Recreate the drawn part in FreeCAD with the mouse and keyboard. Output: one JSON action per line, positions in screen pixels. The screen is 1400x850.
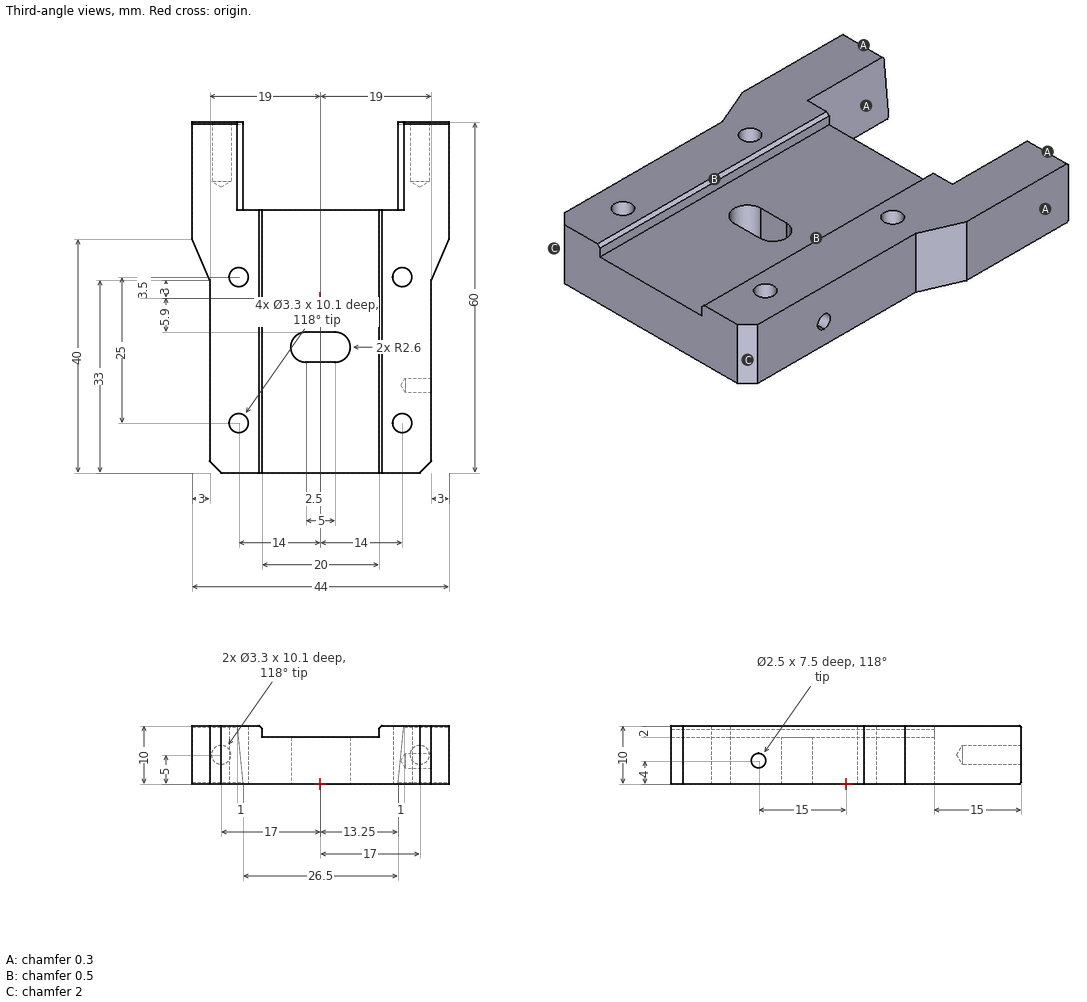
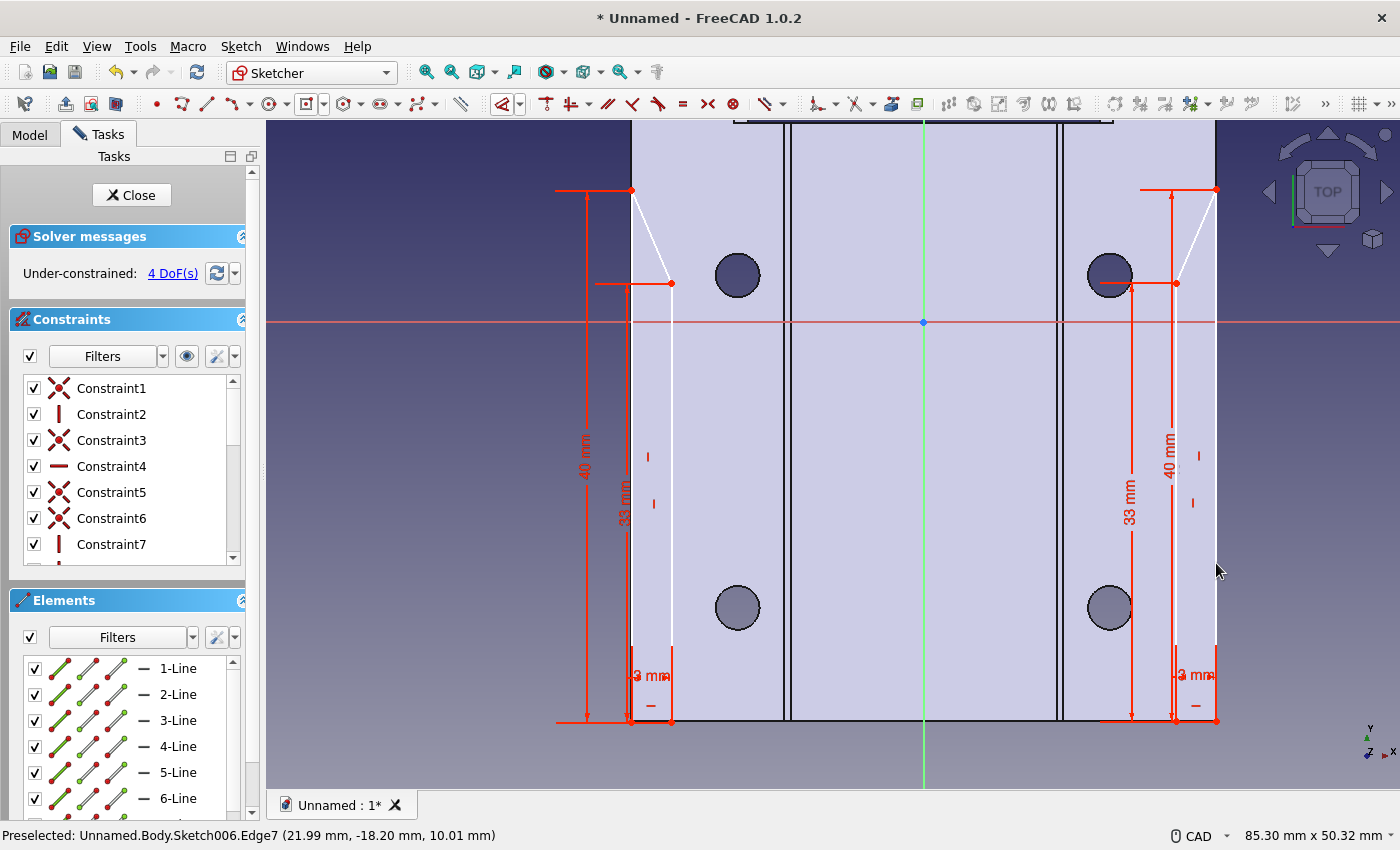
{"action": "left_click", "coordinate": [672, 284]}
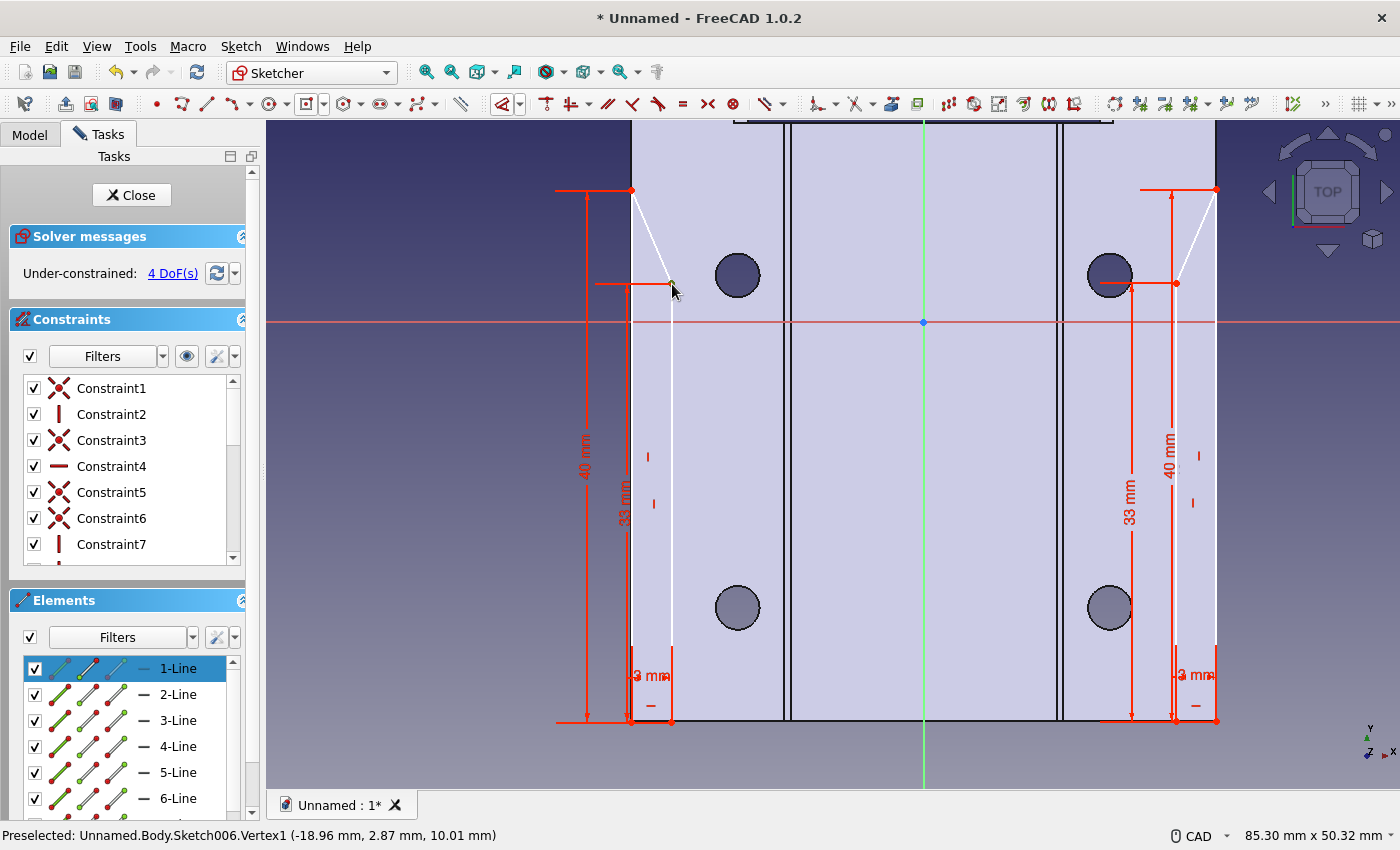
{"action": "key", "text": "i"}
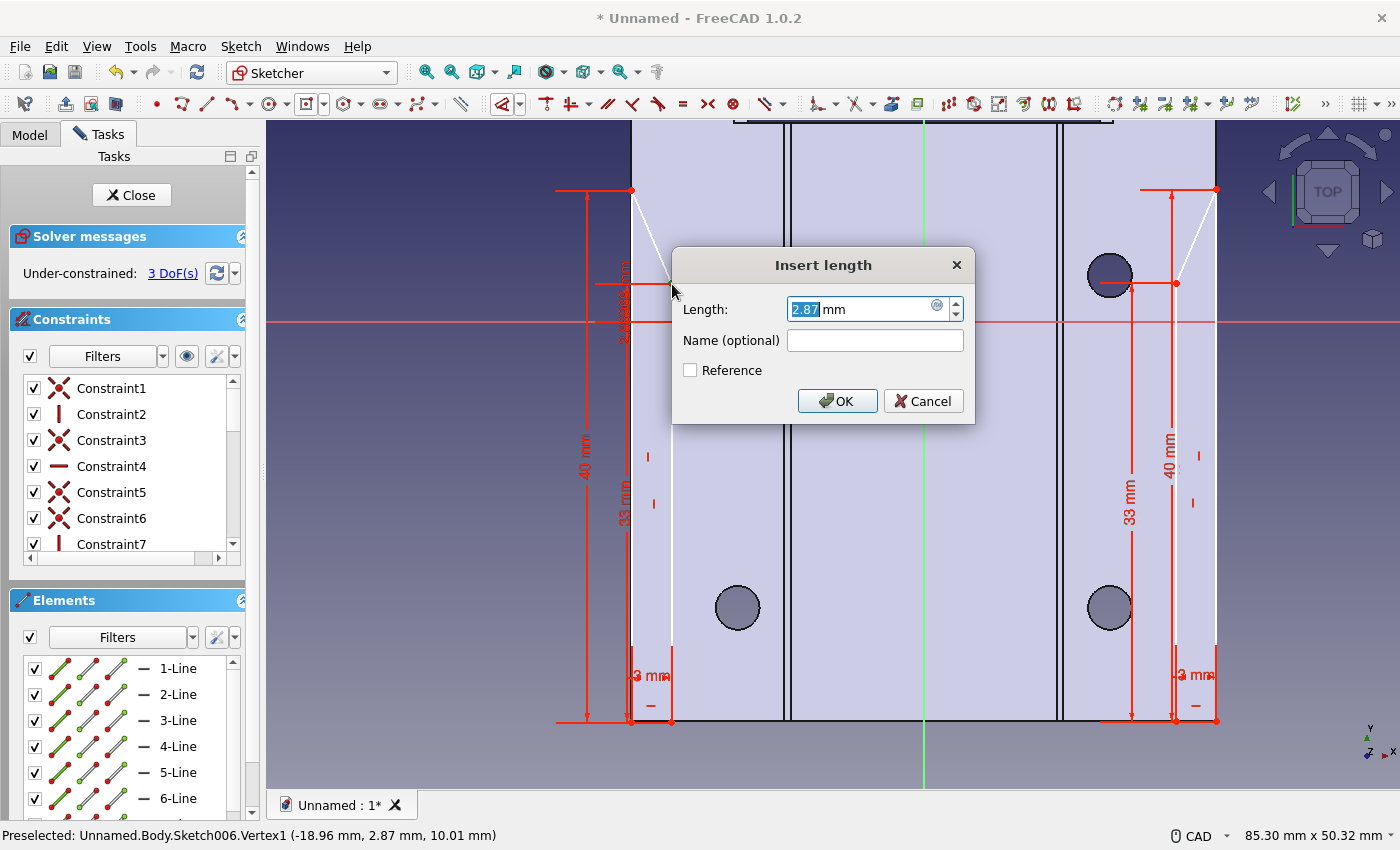
{"action": "type", "text": "3"}
{"action": "key", "text": "Return"}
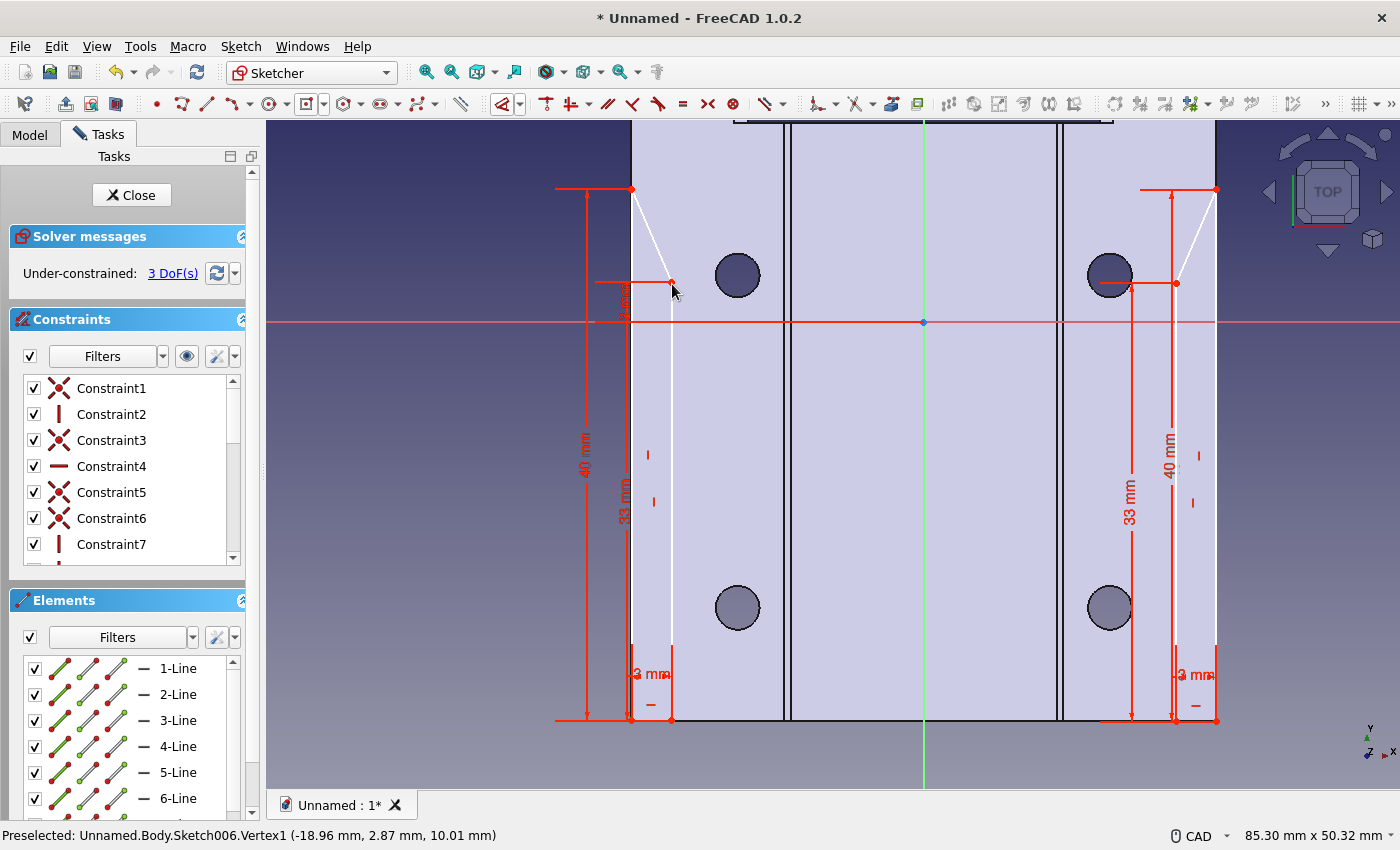
{"action": "left_click", "coordinate": [1176, 283]}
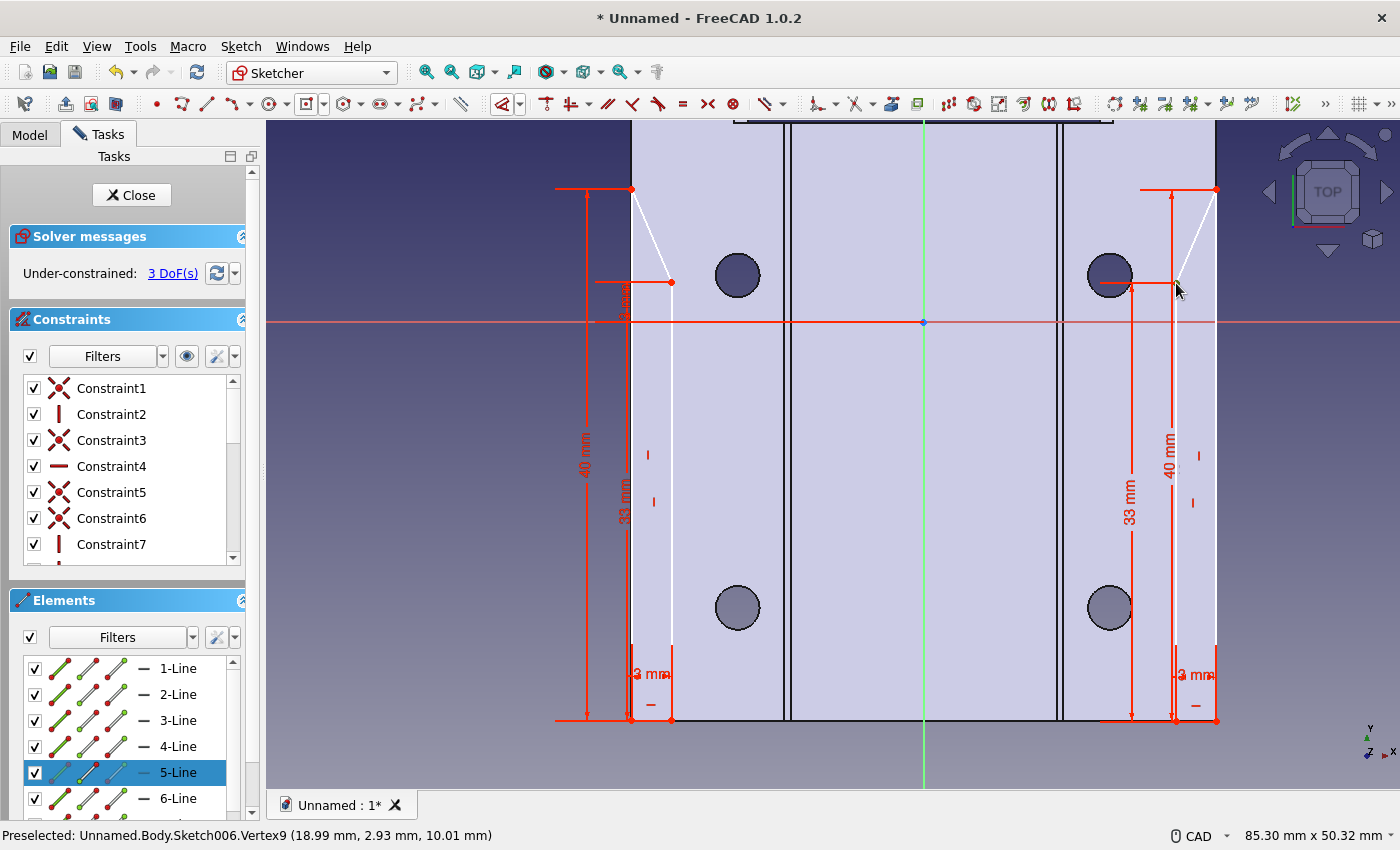
{"action": "left_click", "coordinate": [520, 104]}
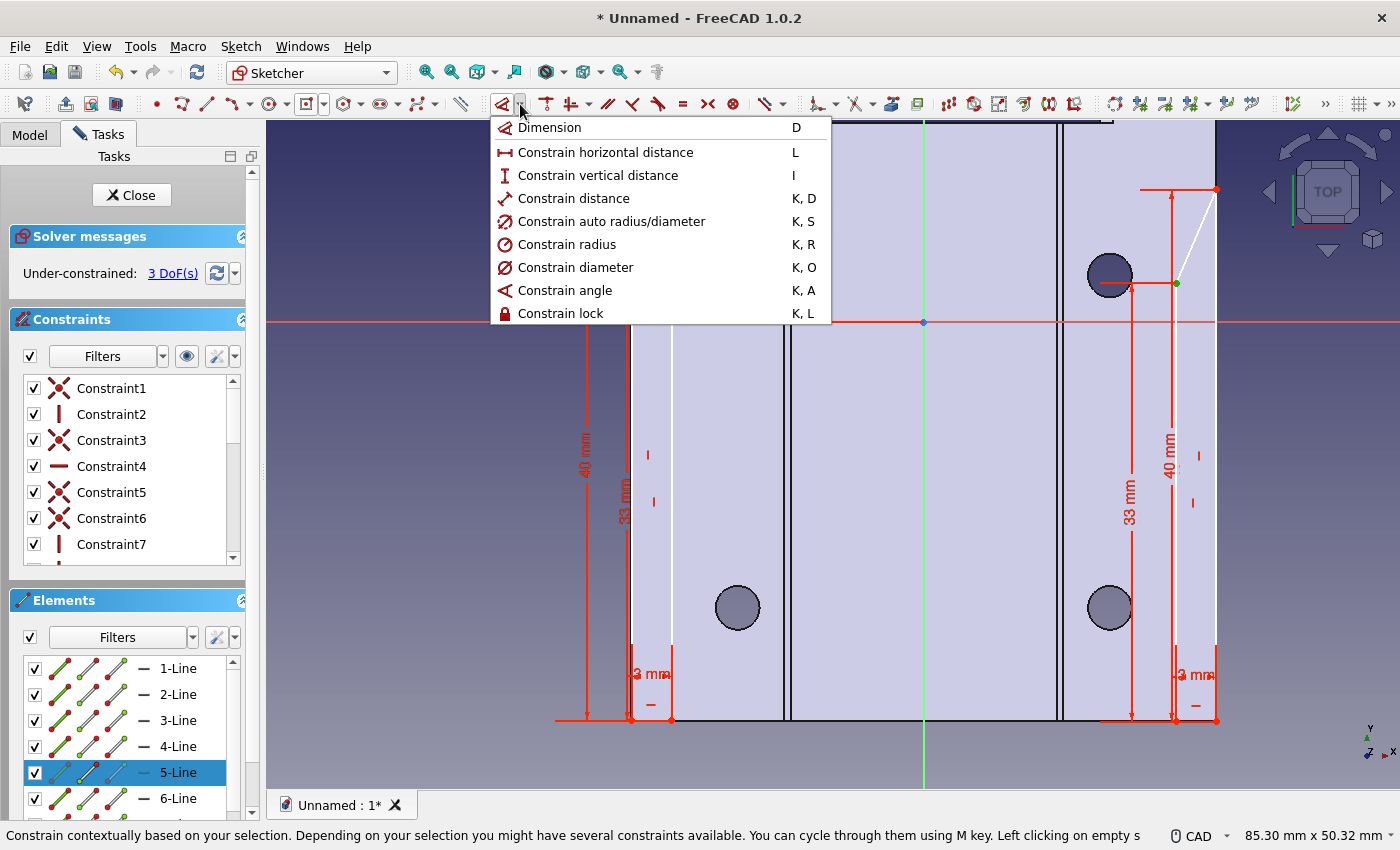
{"action": "left_click", "coordinate": [661, 176]}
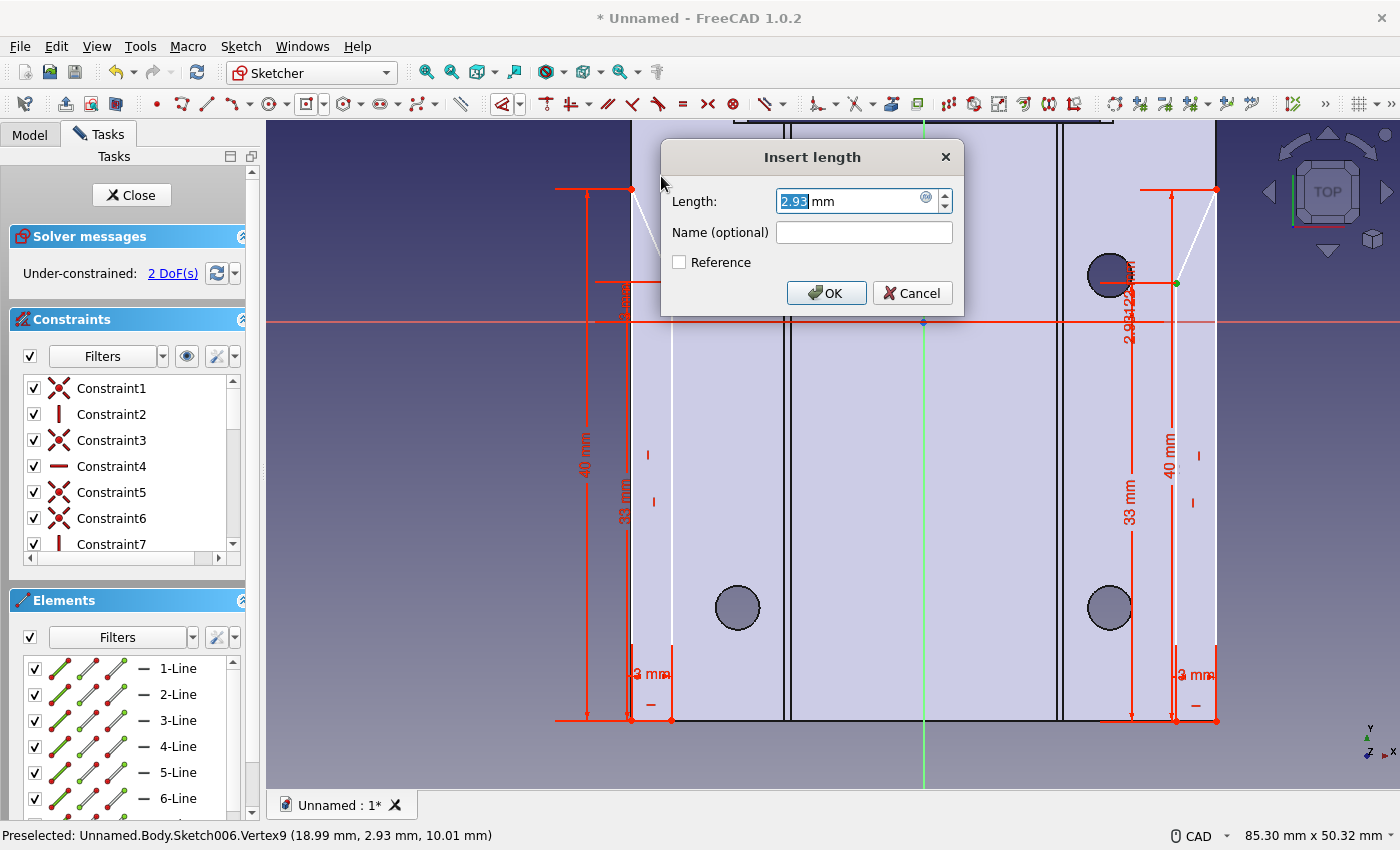
{"action": "type", "text": "3"}
{"action": "key", "text": "Return"}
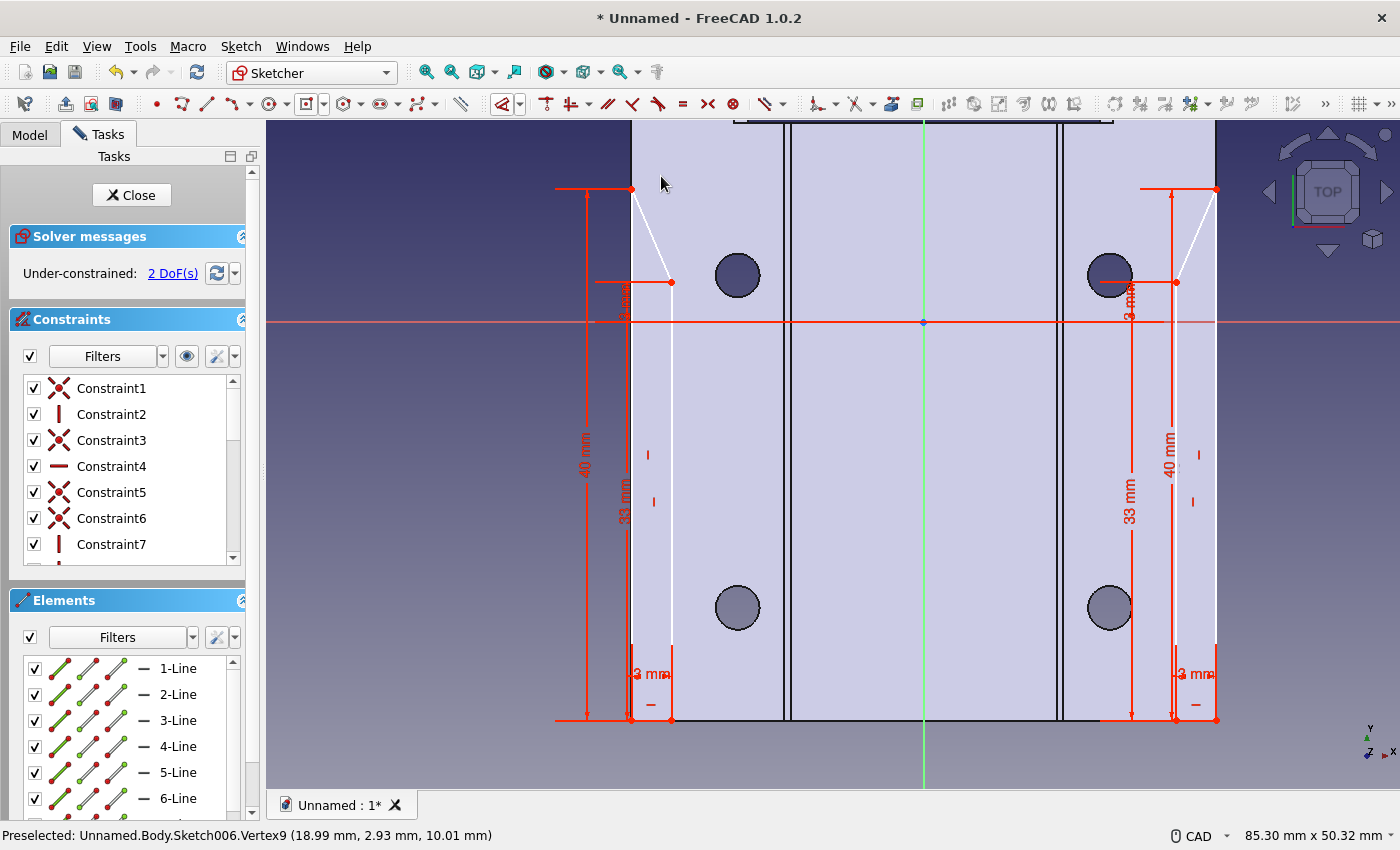
{"action": "left_click", "coordinate": [672, 282]}